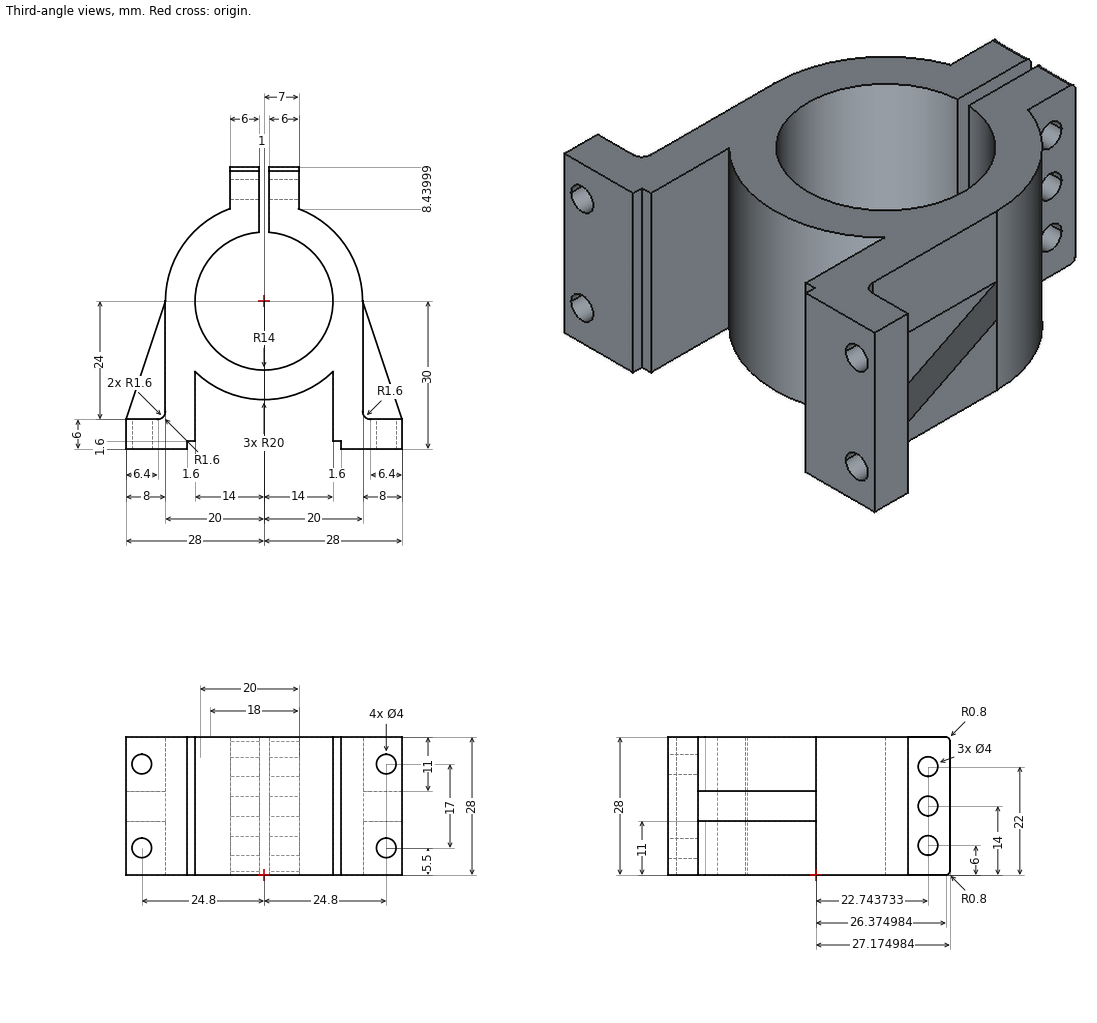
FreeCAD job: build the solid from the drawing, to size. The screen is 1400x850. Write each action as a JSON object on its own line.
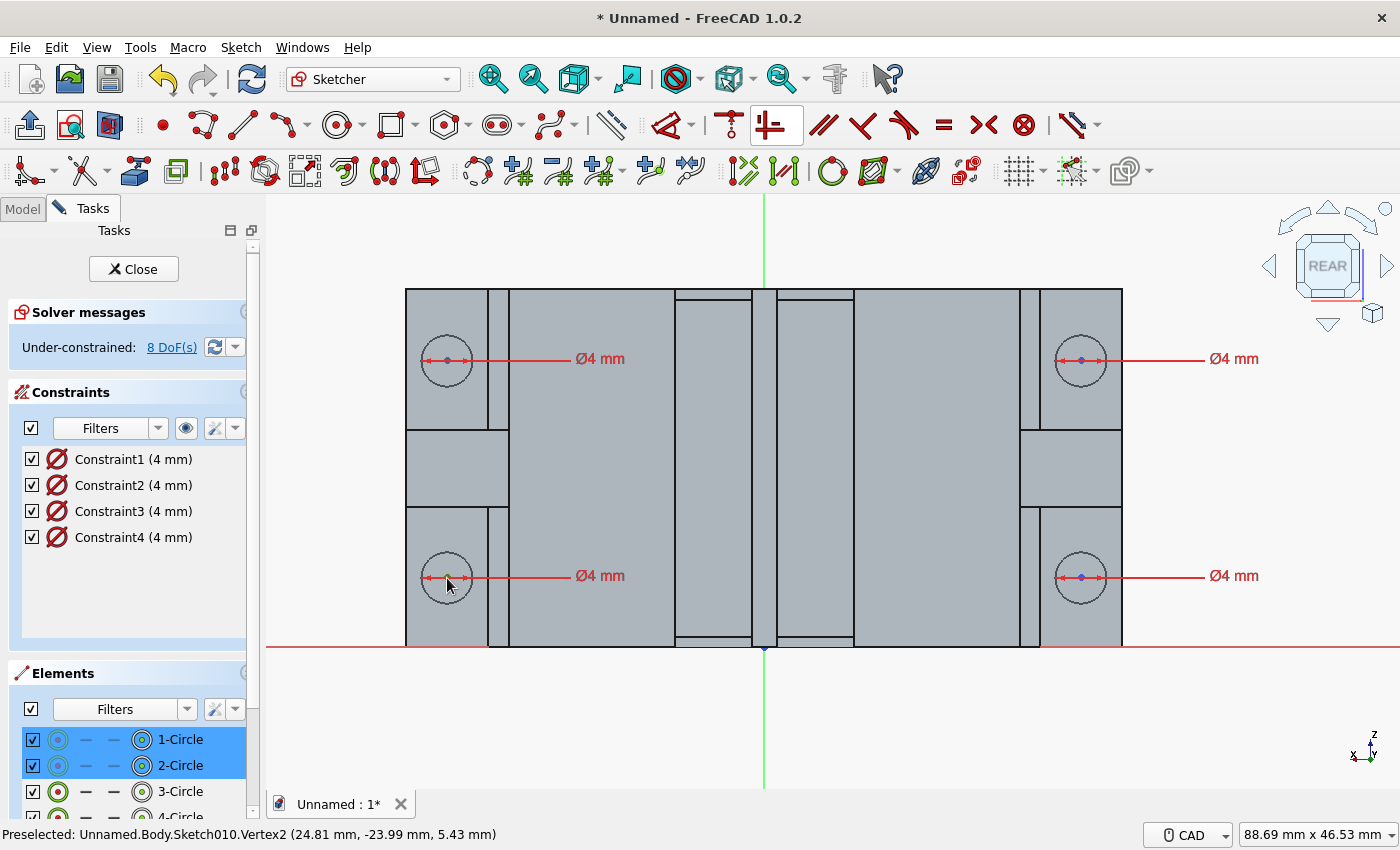
{"action": "left_click", "coordinate": [798, 126]}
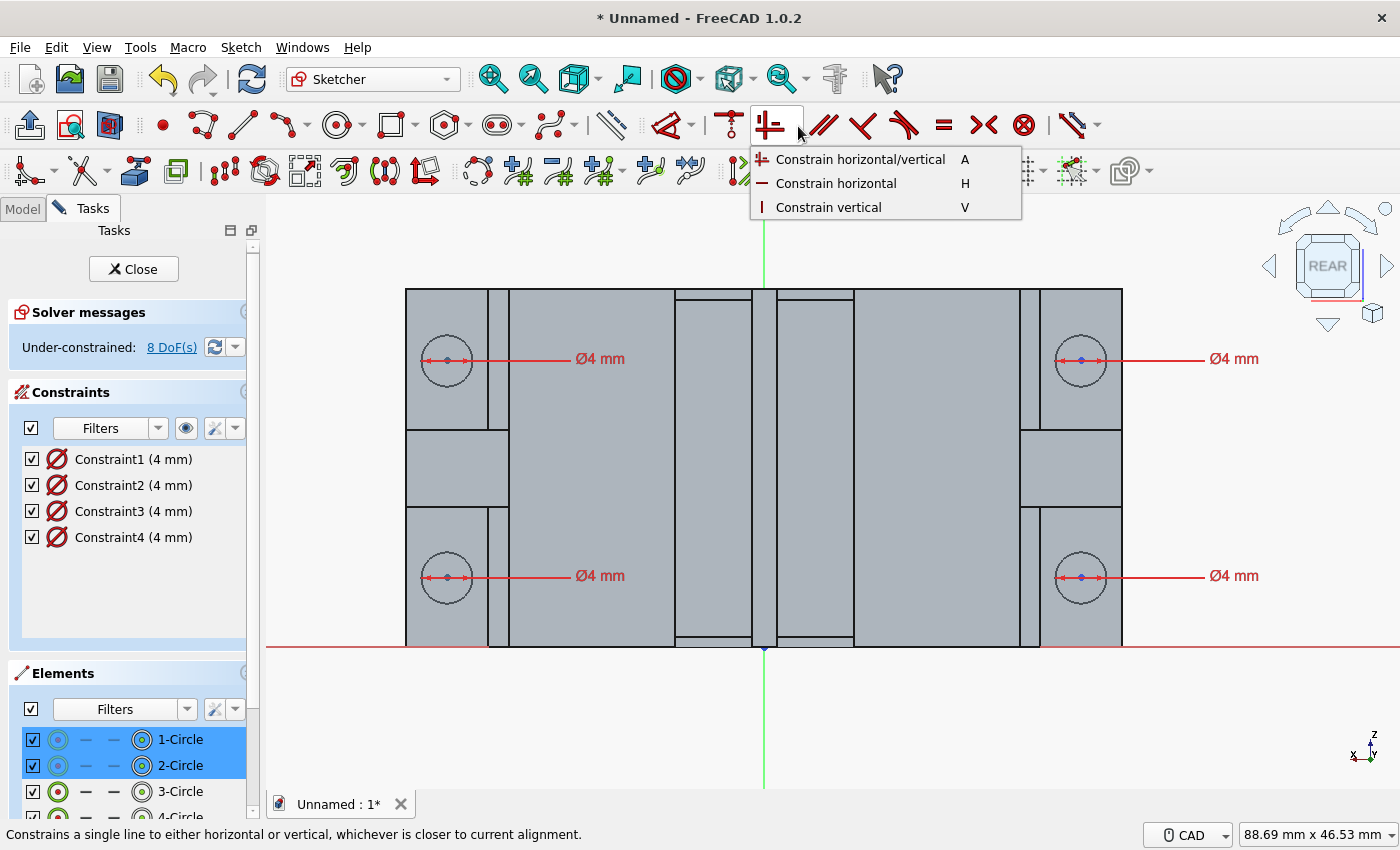
{"action": "left_click", "coordinate": [886, 207]}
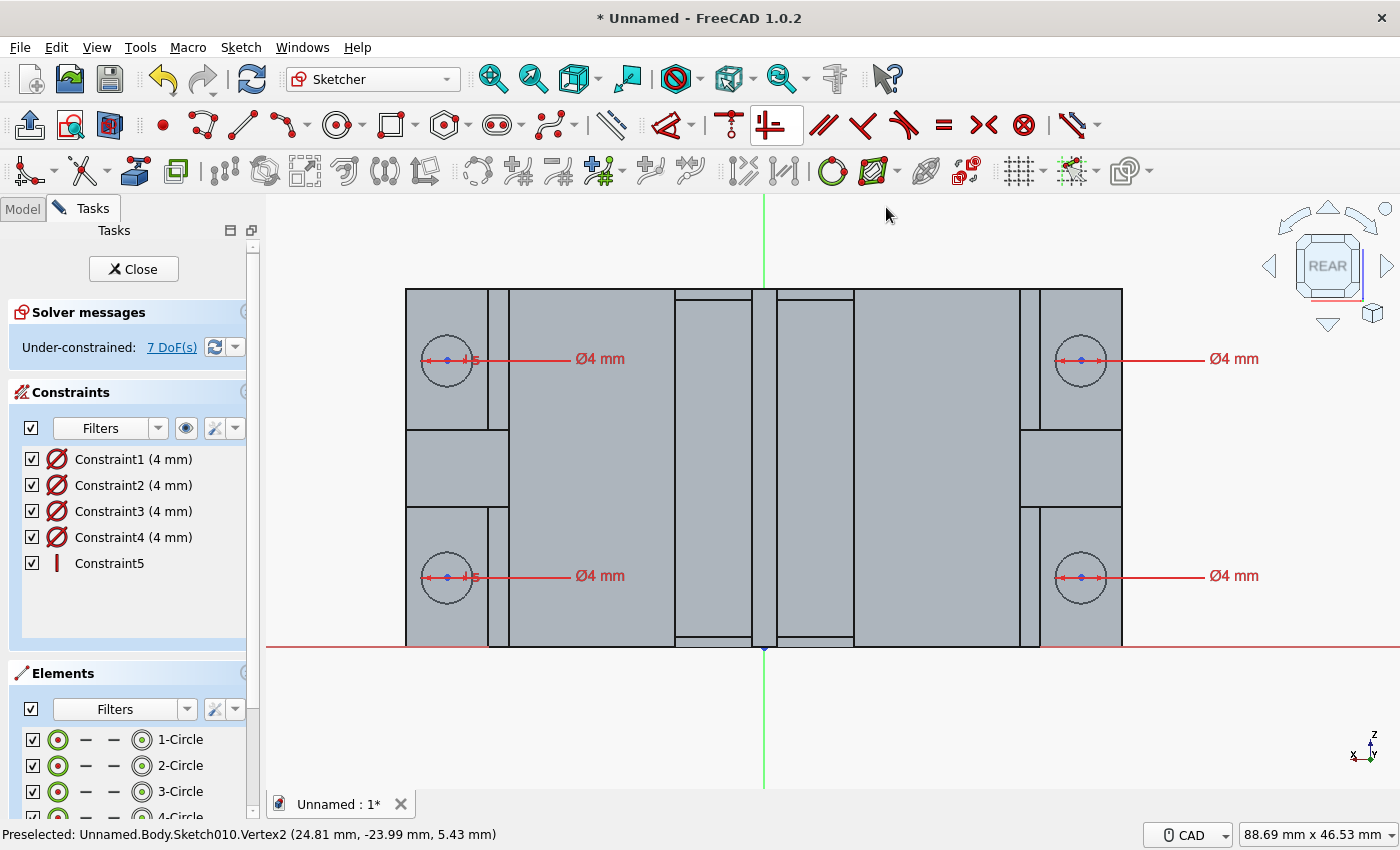
{"action": "left_click", "coordinate": [447, 578]}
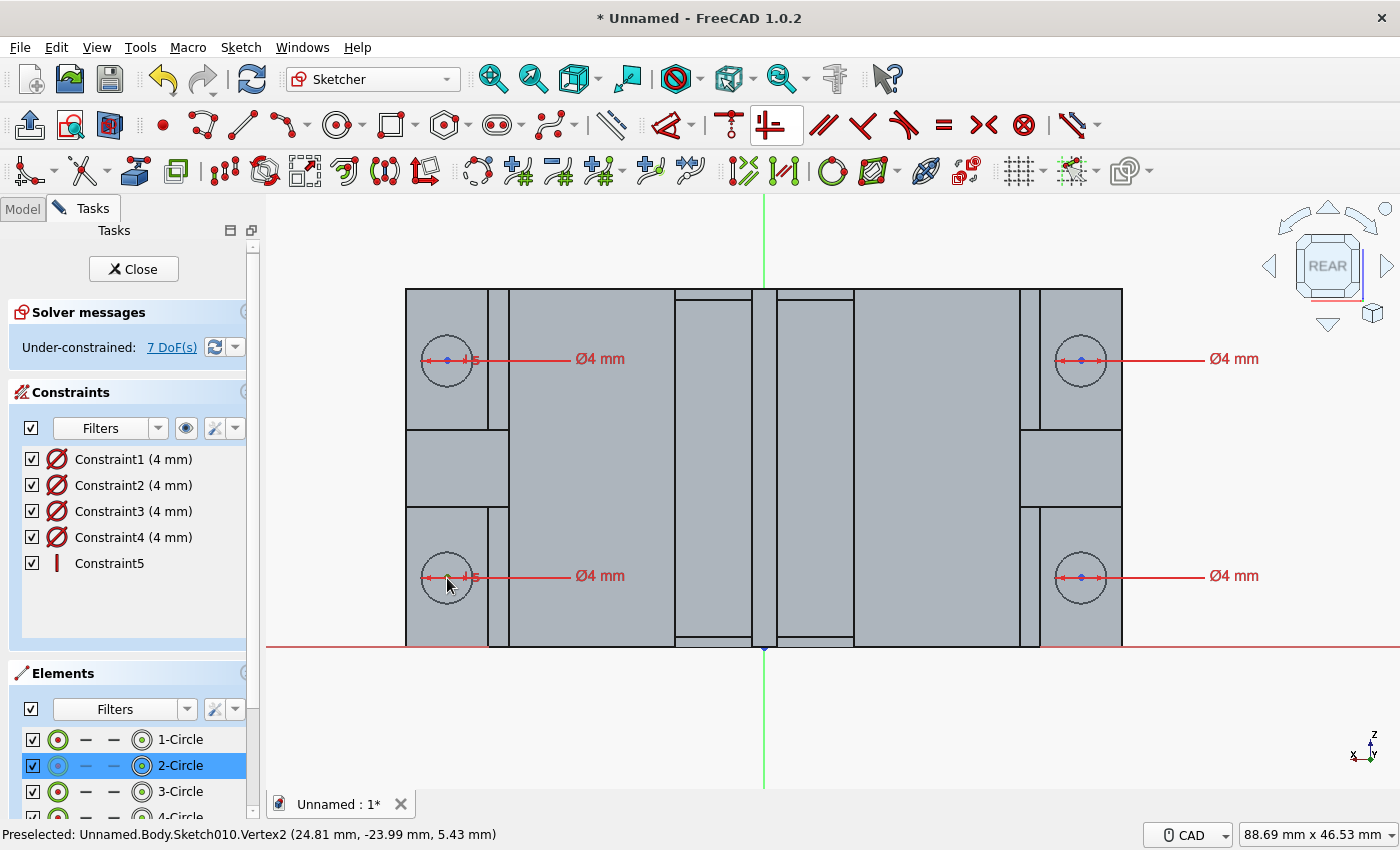
{"action": "left_click", "coordinate": [1081, 578]}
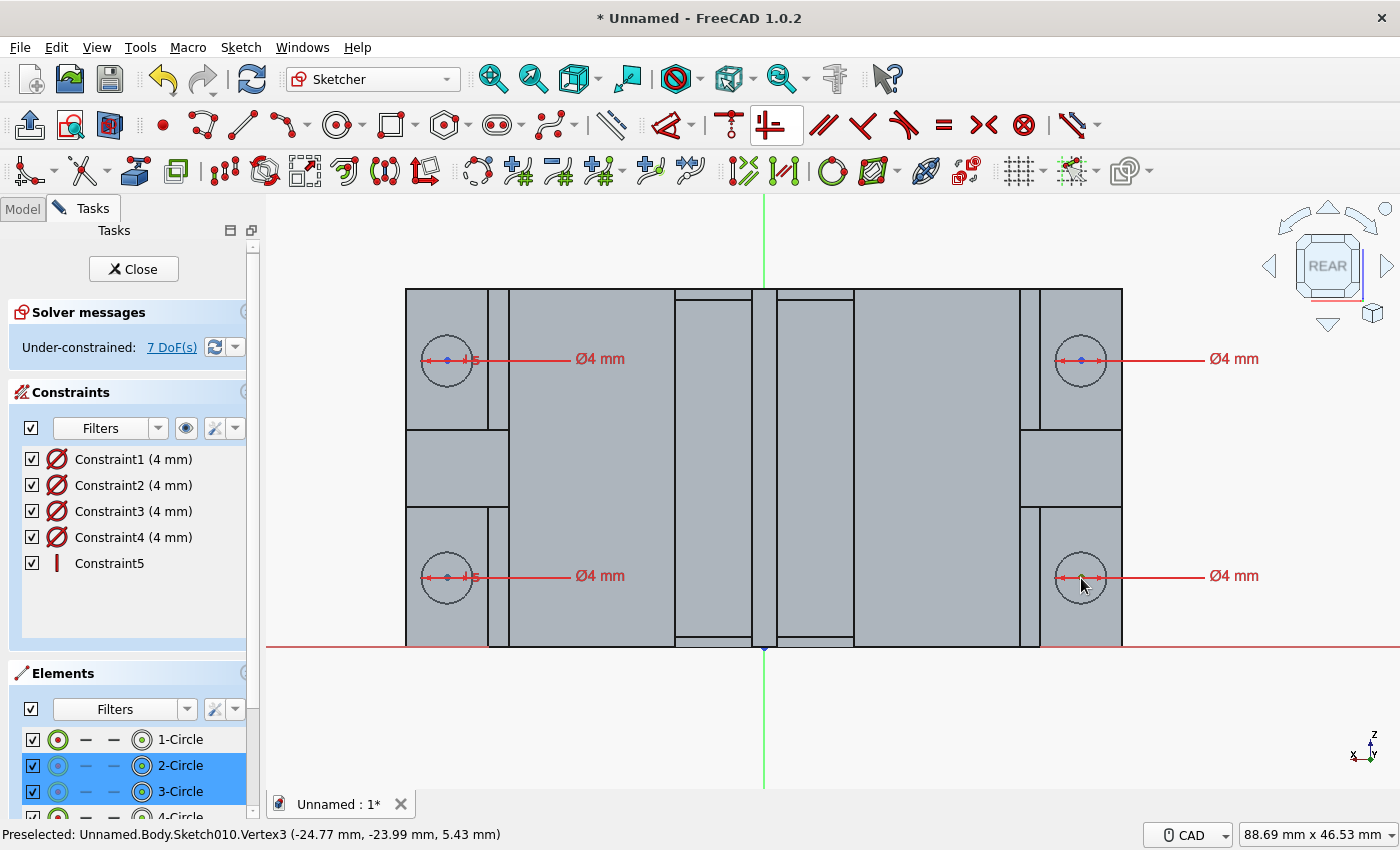
{"action": "left_click", "coordinate": [798, 126]}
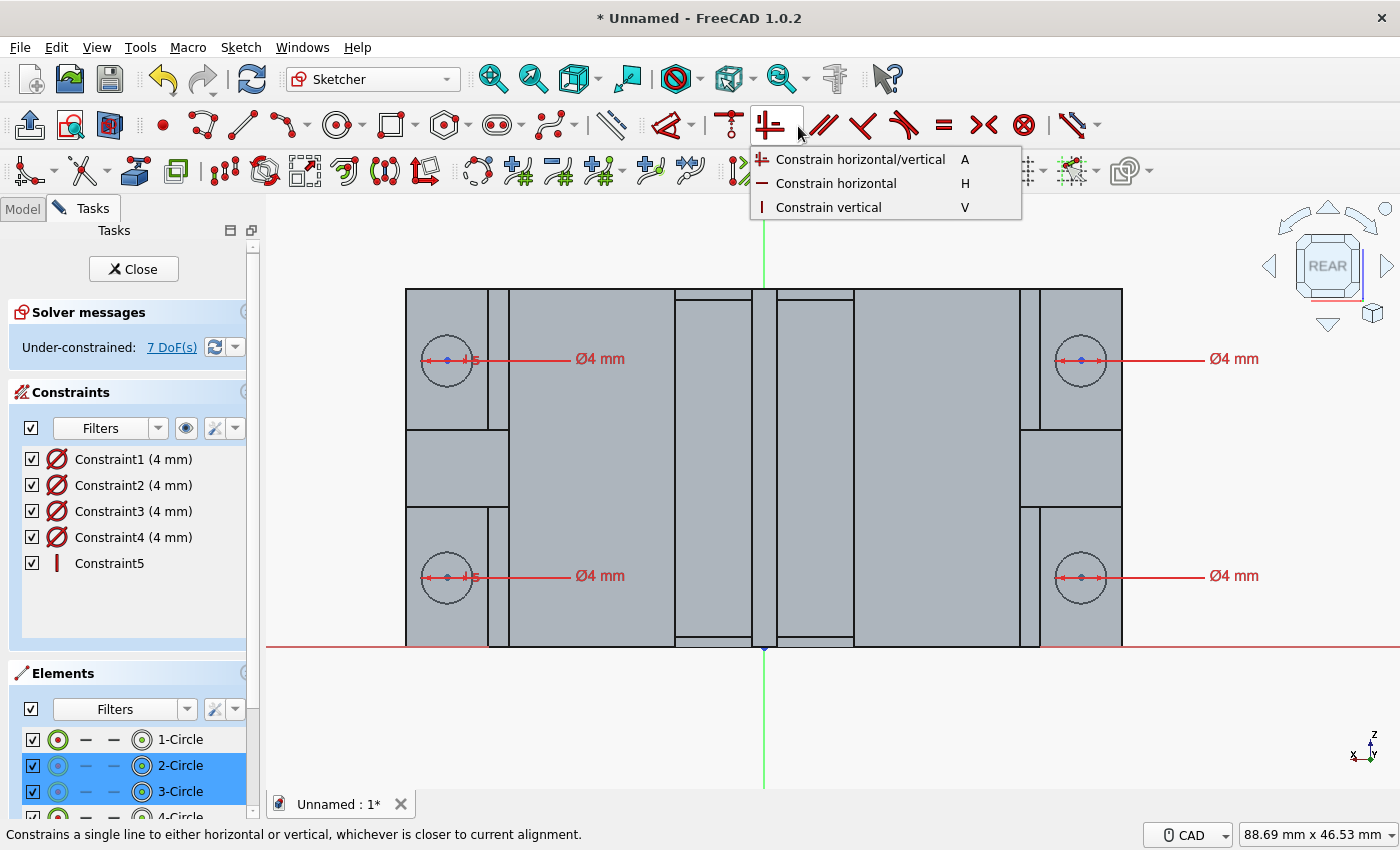
{"action": "left_click", "coordinate": [886, 183]}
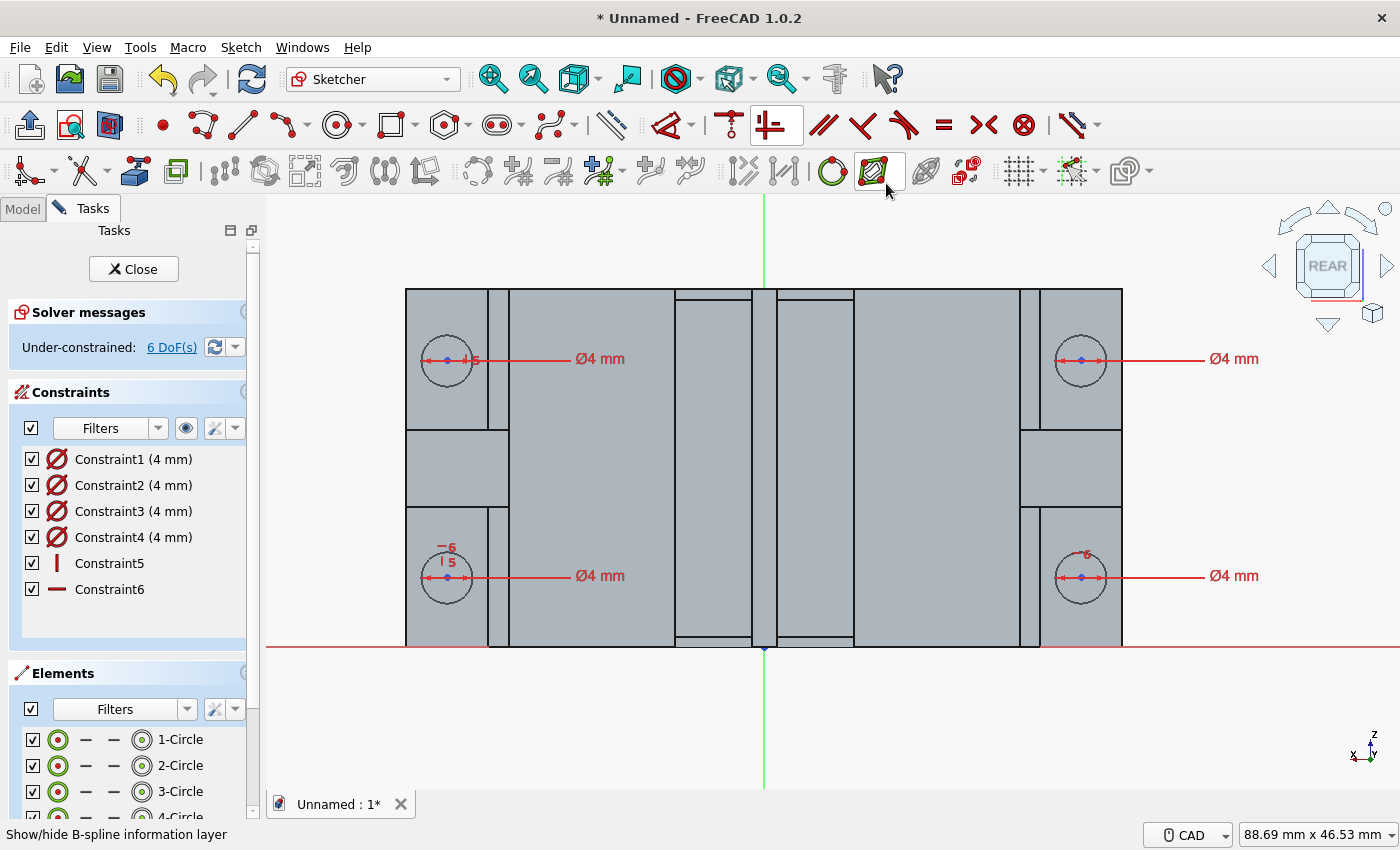
{"action": "left_click", "coordinate": [1081, 578]}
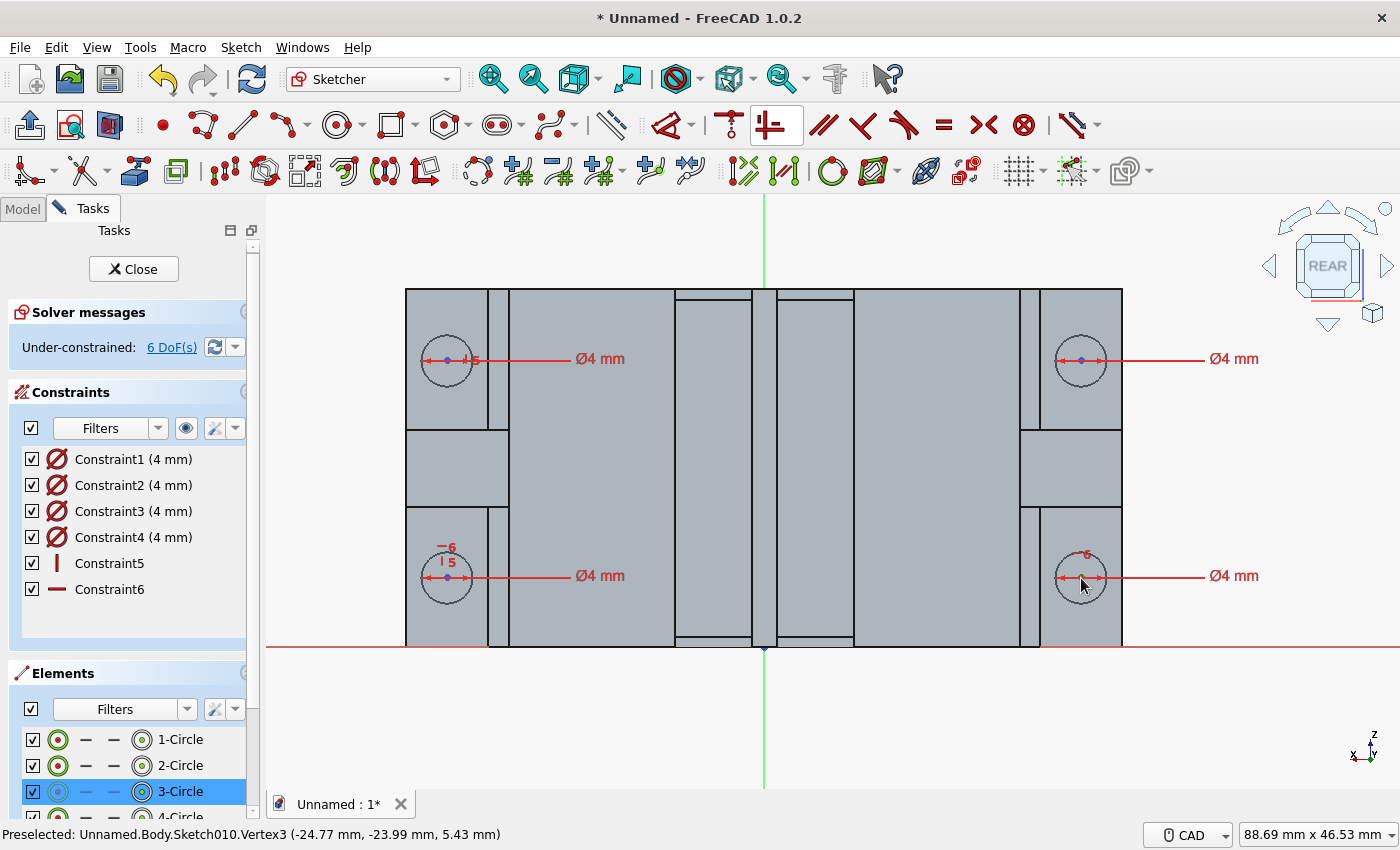
{"action": "left_click", "coordinate": [1081, 361]}